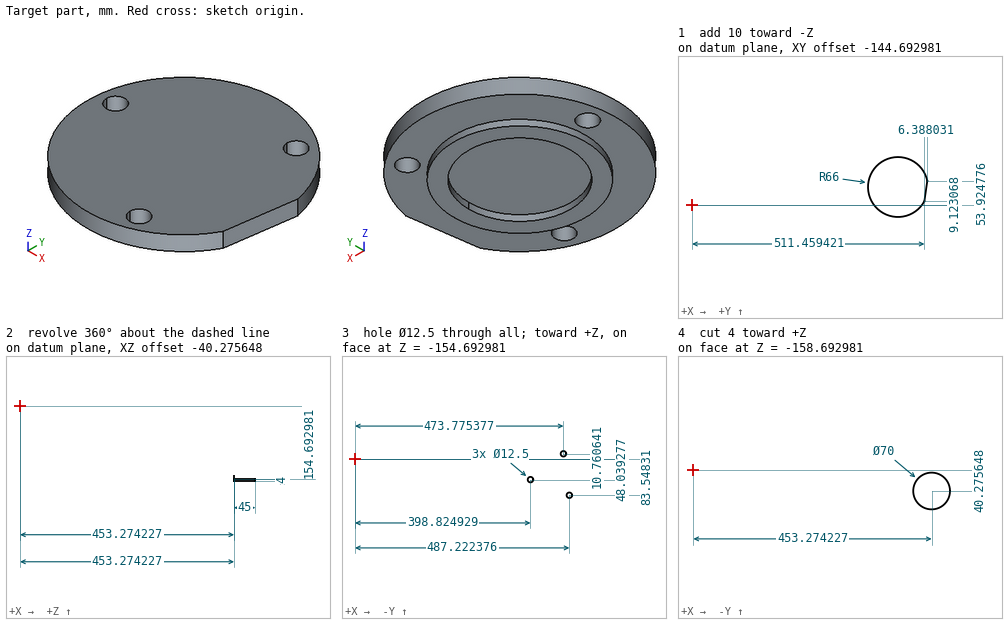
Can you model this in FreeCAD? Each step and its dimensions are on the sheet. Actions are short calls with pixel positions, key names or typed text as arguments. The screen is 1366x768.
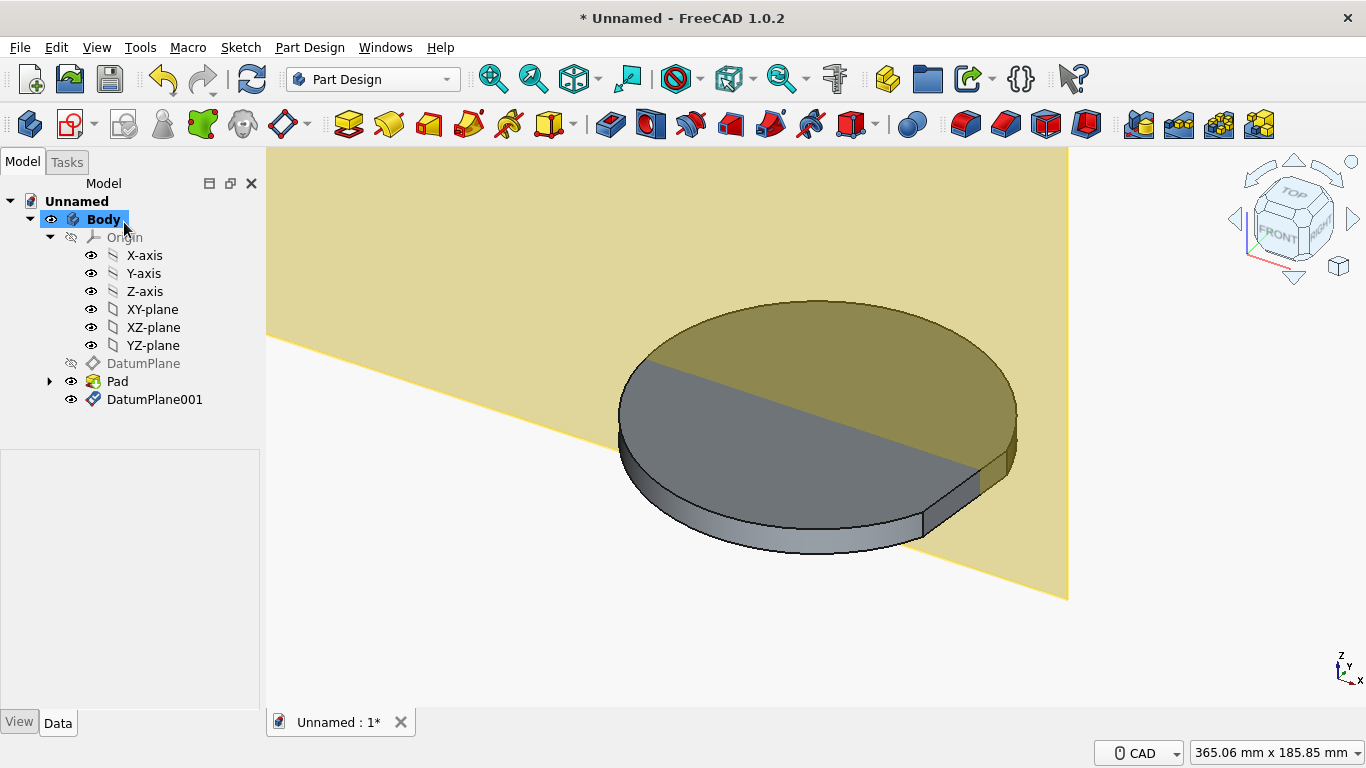
click(116, 399)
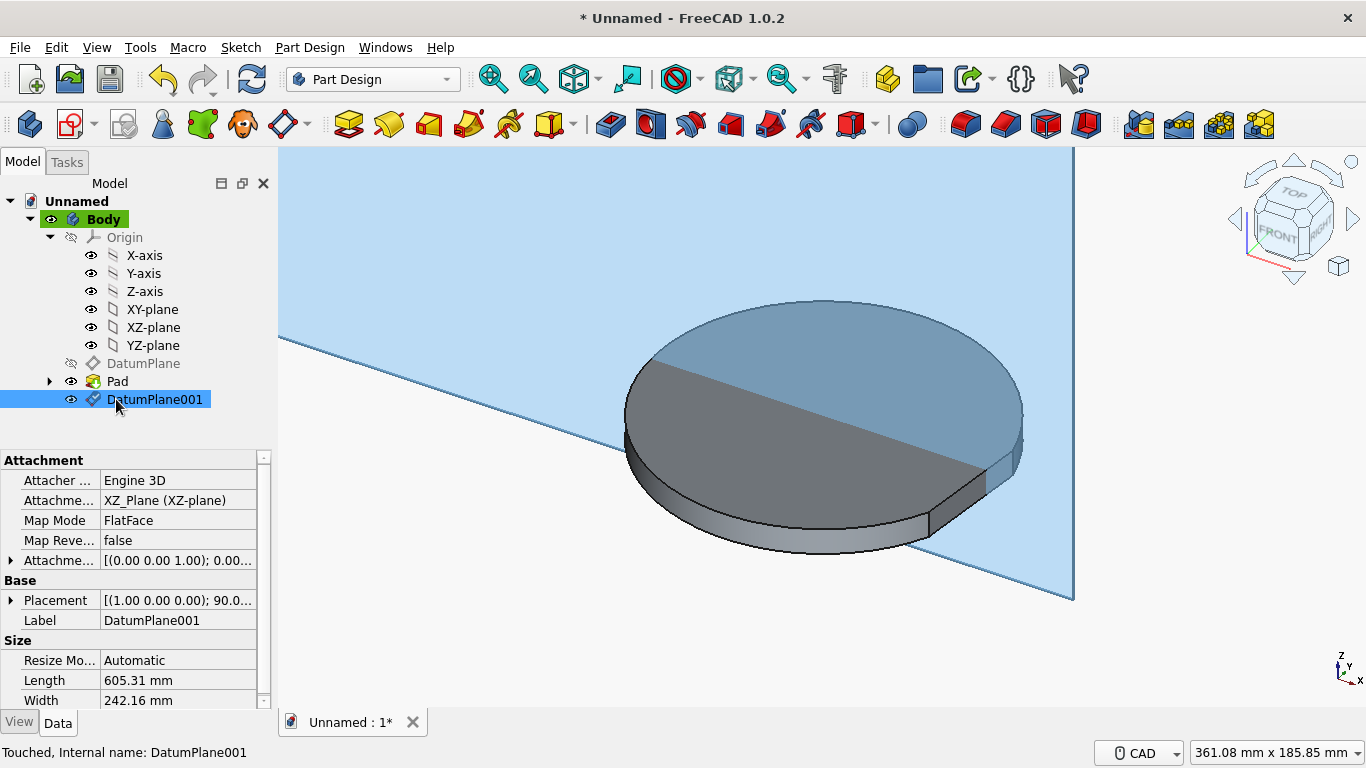
click(70, 124)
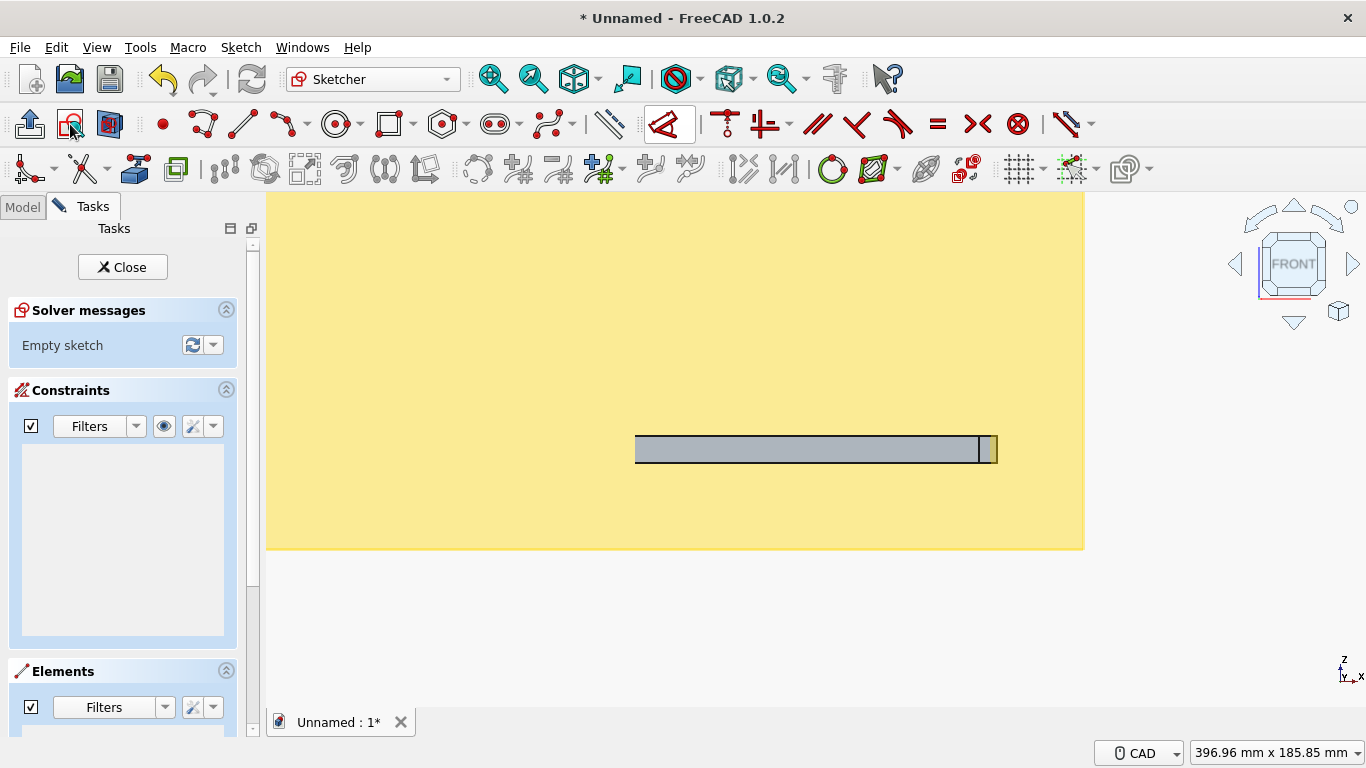
click(110, 124)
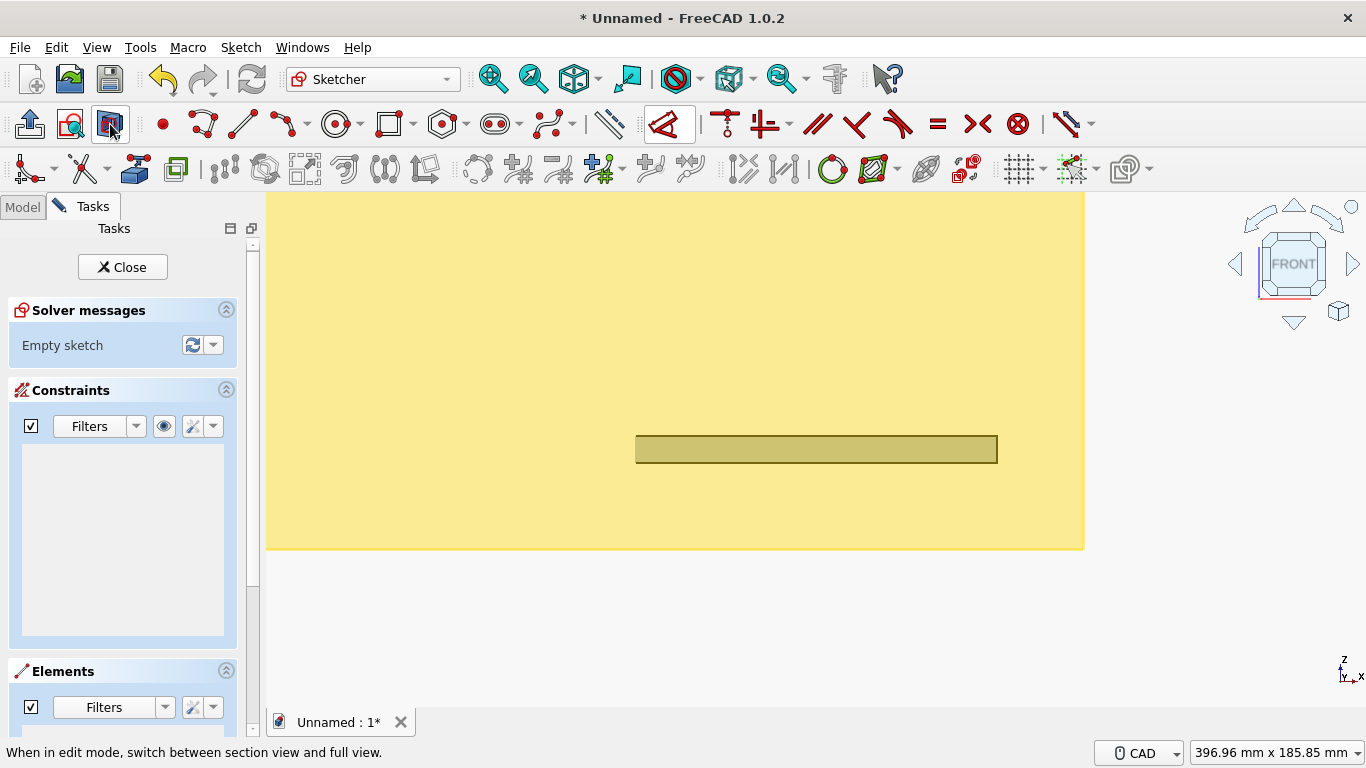
scroll(914, 461, up, 8)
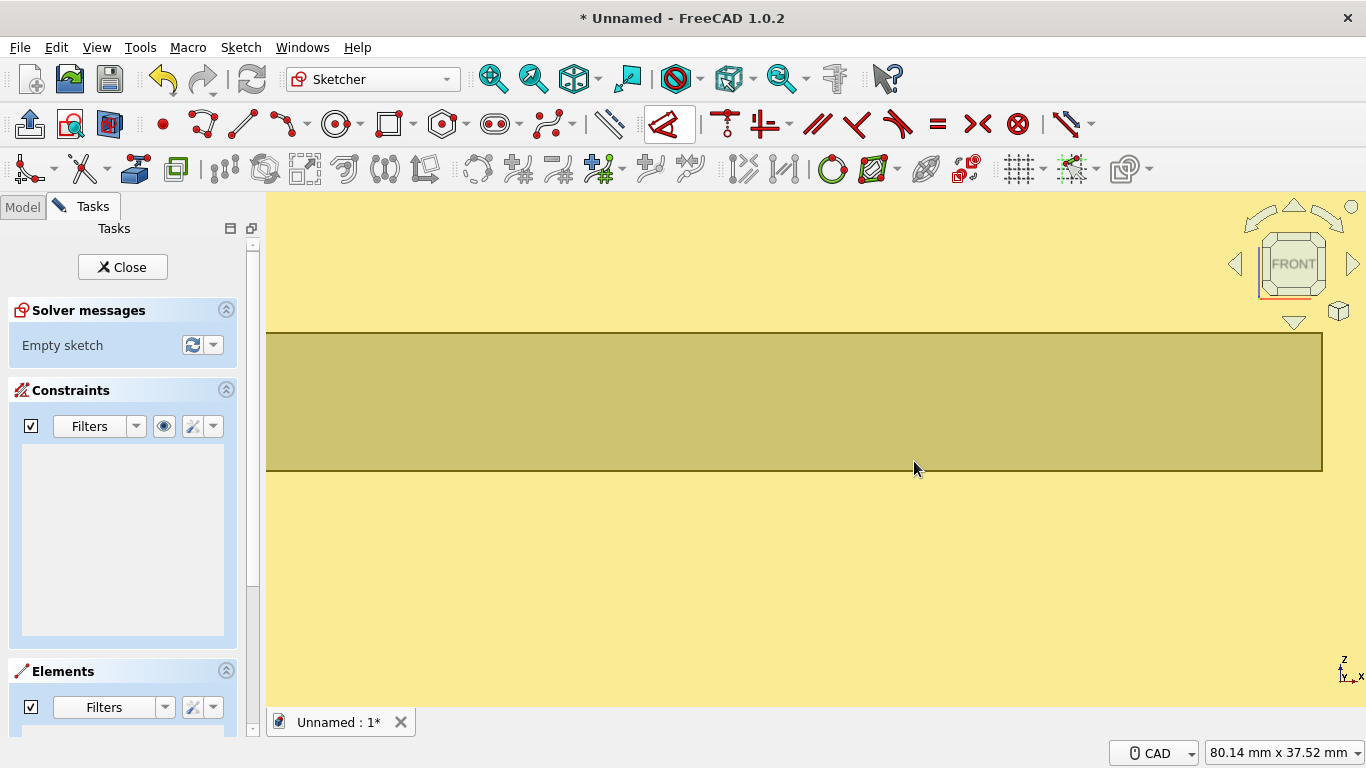
key(g)
key(r)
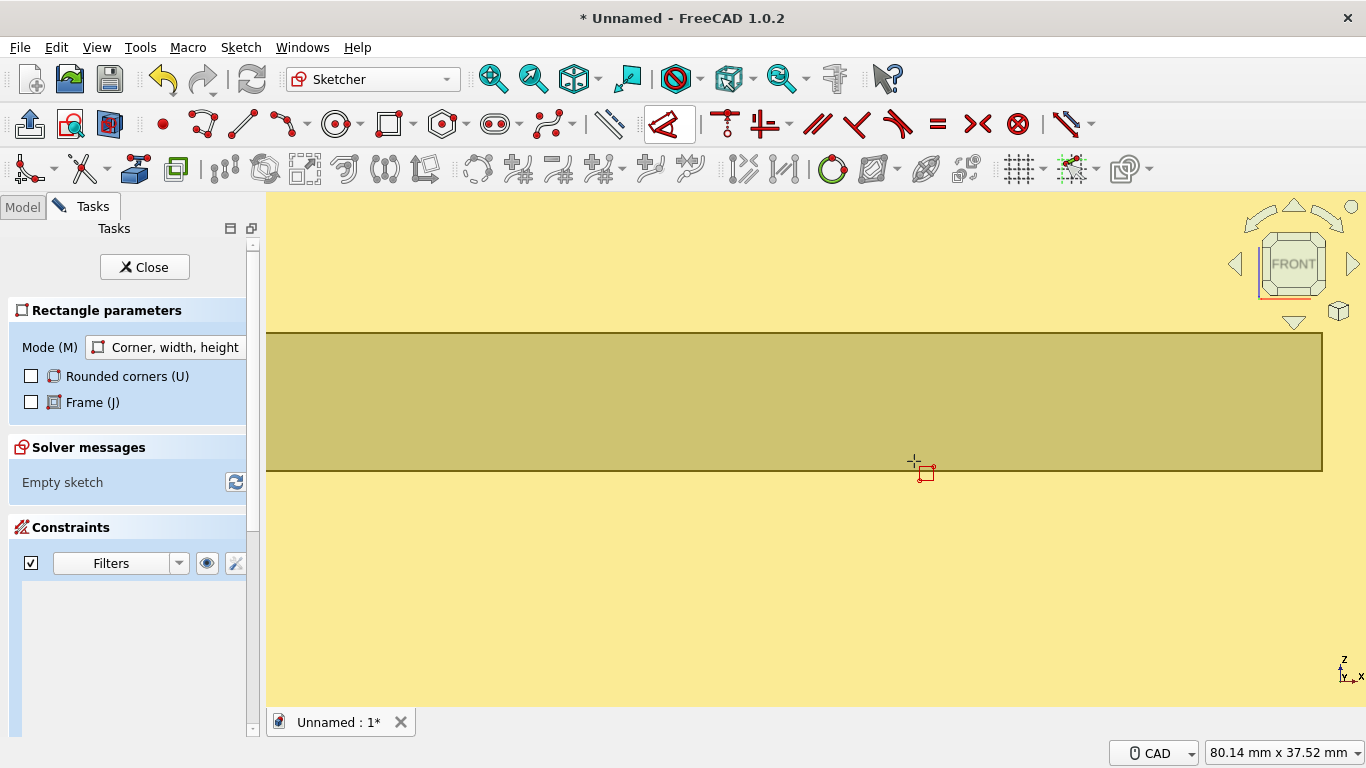
click(436, 471)
move(1053, 525)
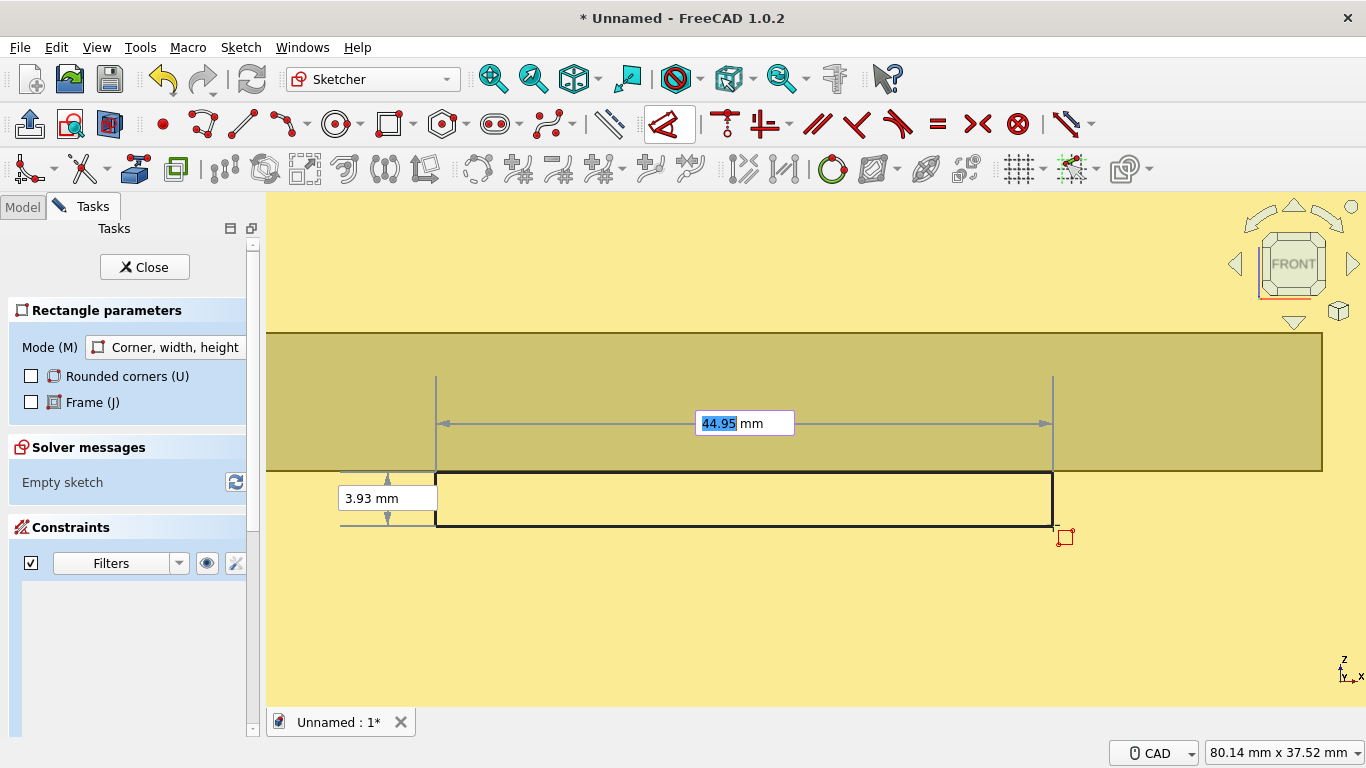
text(45)
key(Tab)
text(4)
key(Return)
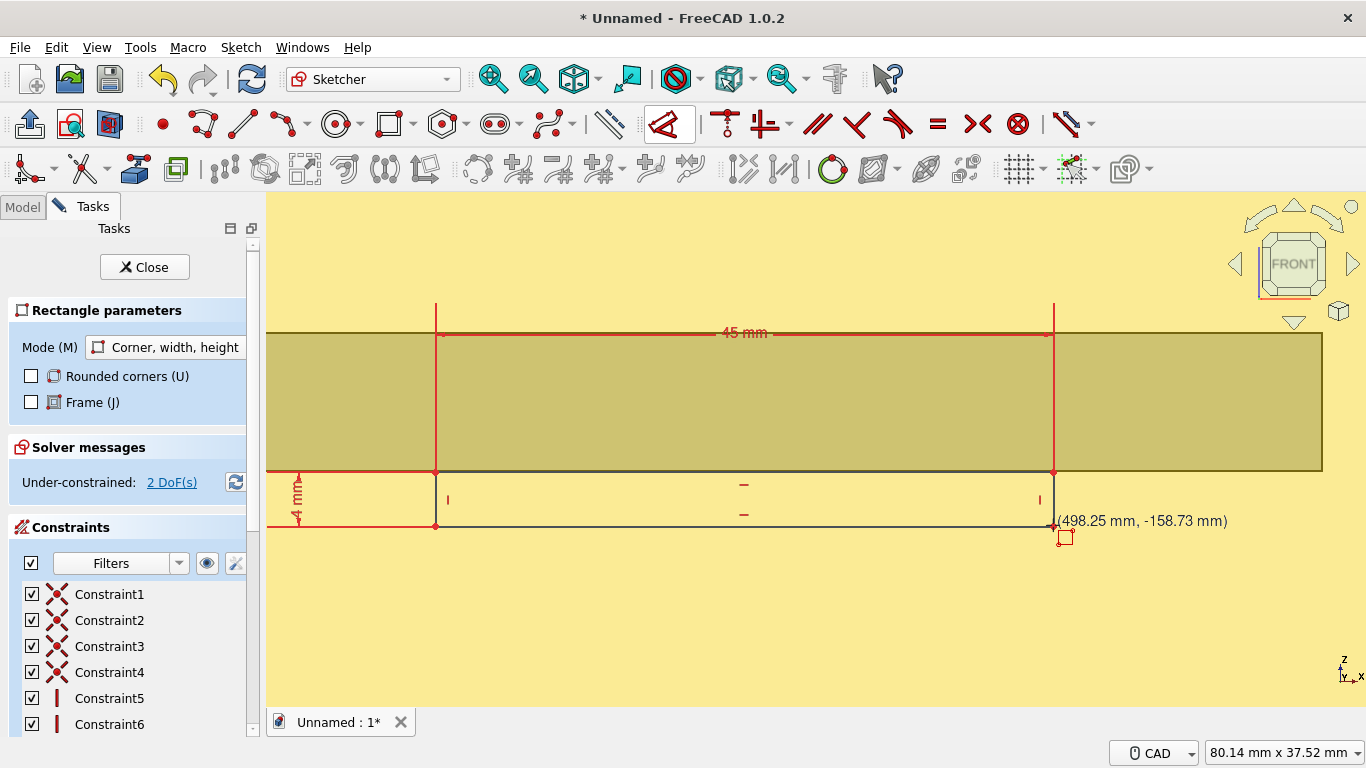
click(244, 124)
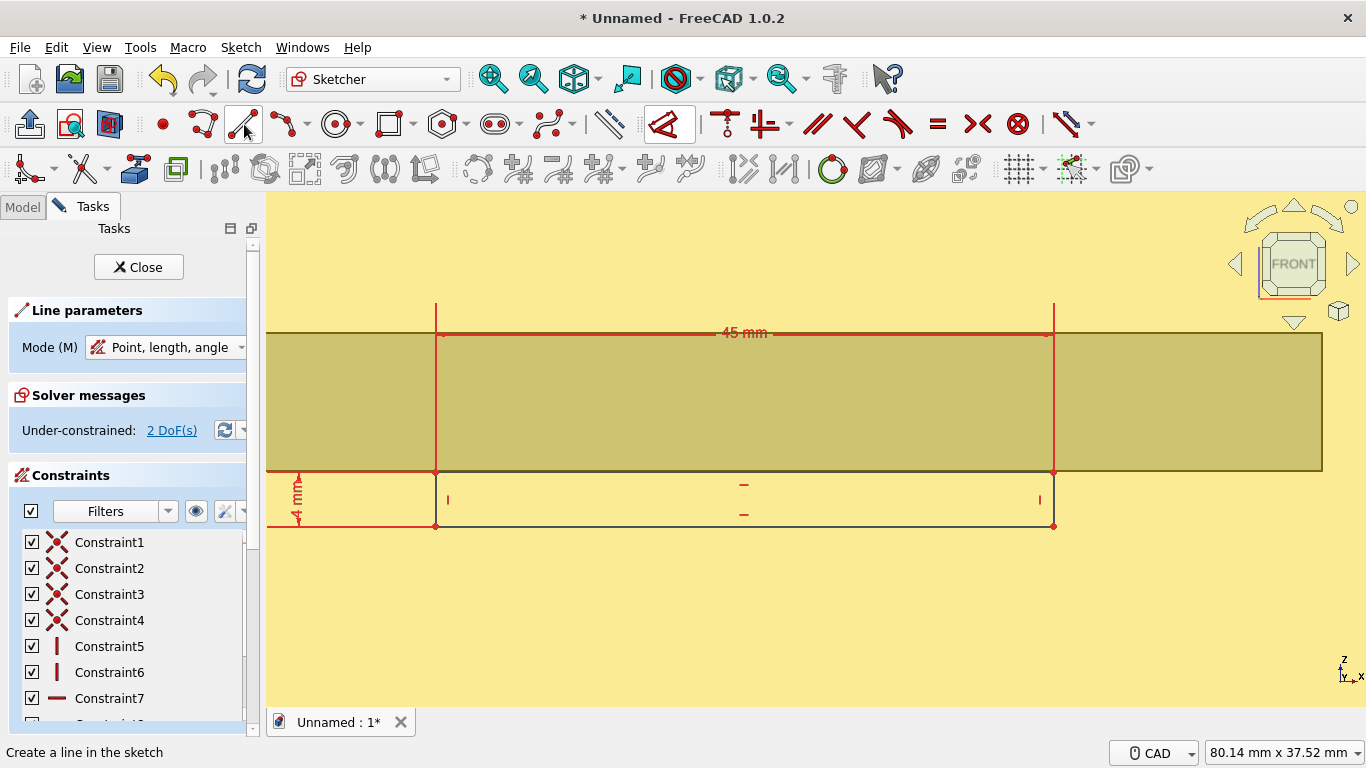
click(436, 446)
click(436, 372)
key(Escape)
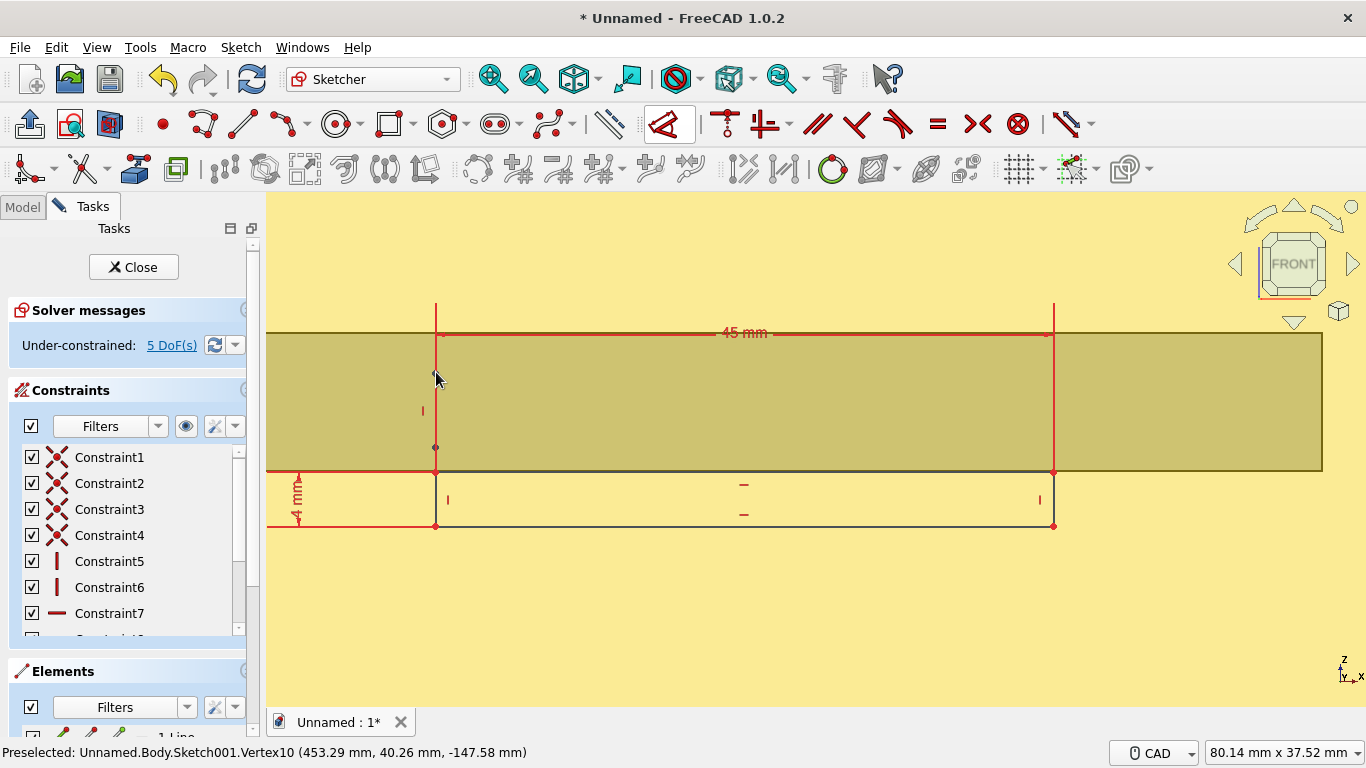
click(436, 425)